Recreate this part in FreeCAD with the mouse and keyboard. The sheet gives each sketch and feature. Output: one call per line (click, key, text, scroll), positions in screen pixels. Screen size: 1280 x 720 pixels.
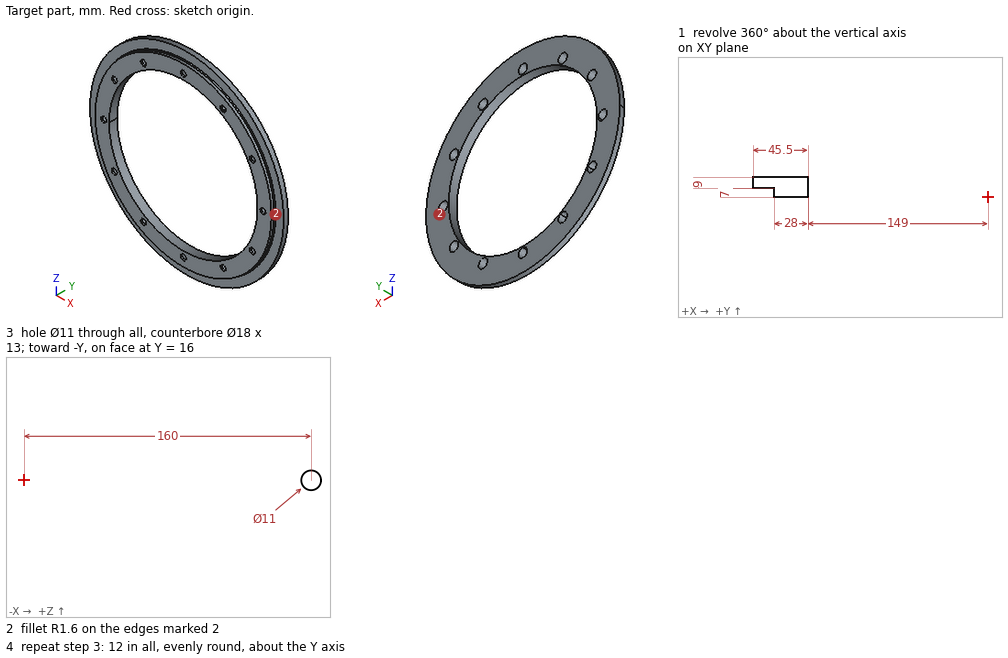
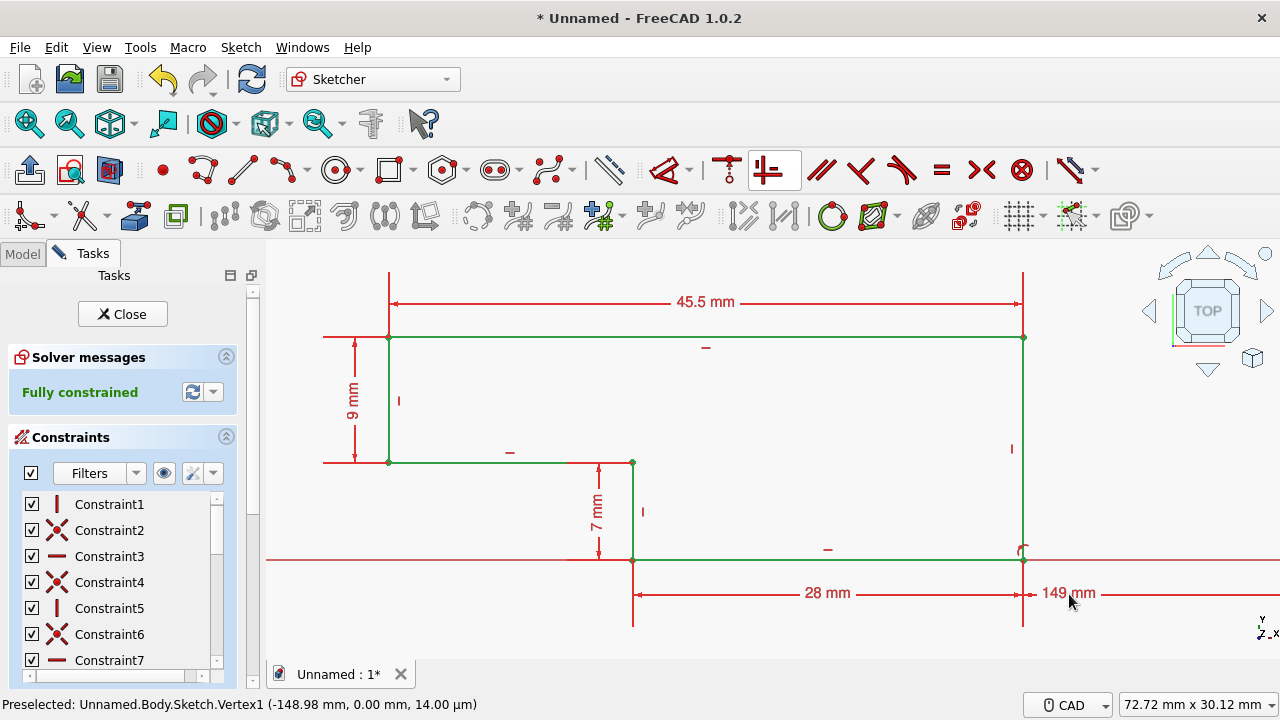
click(123, 314)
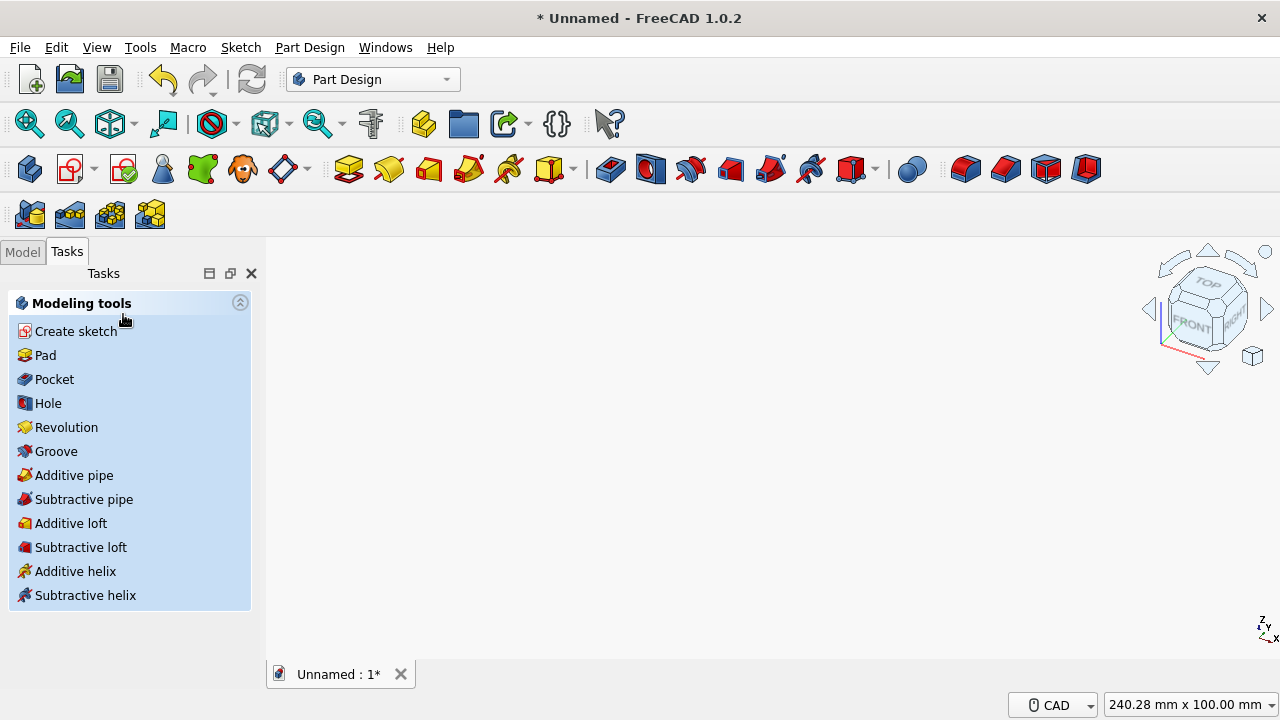
click(390, 170)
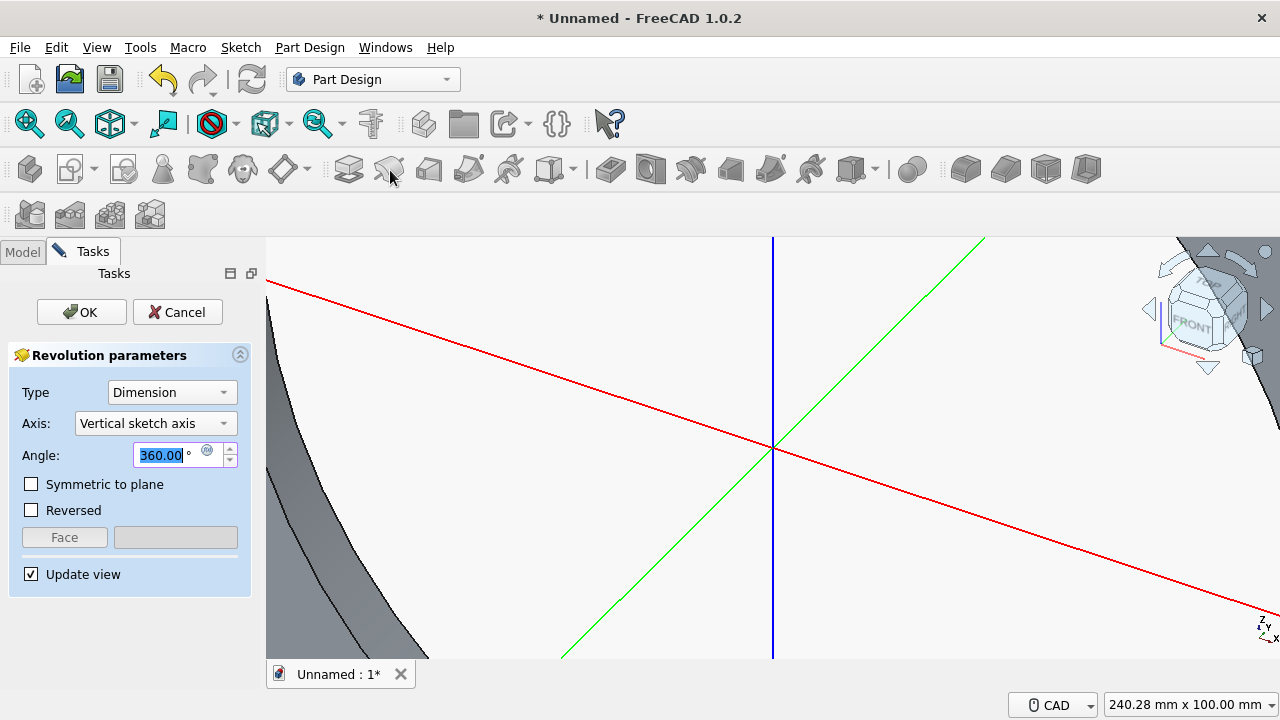
click(82, 312)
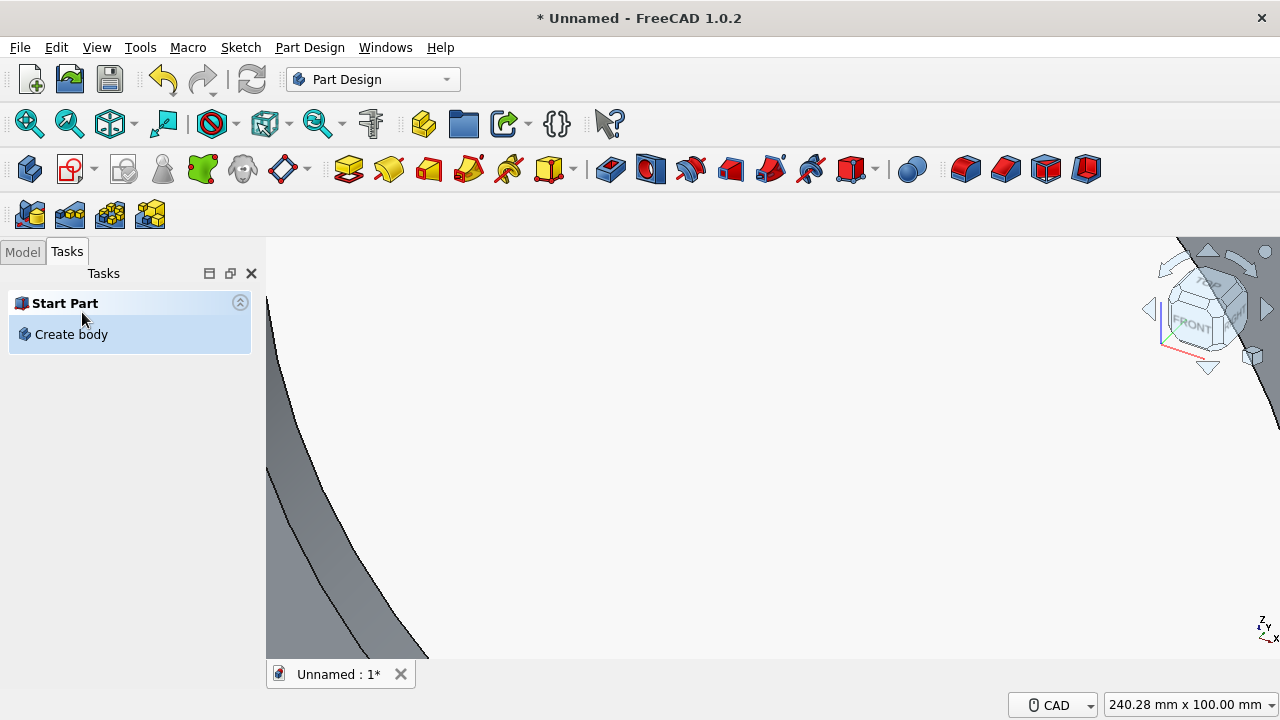
click(30, 124)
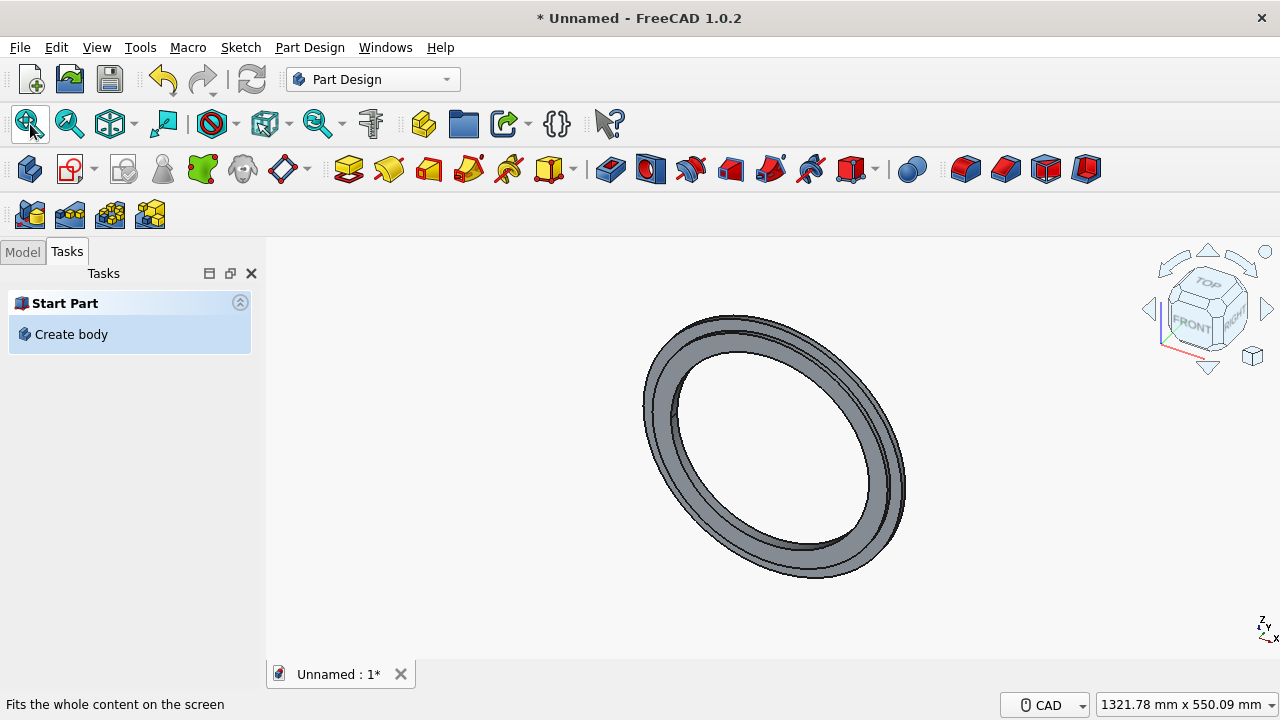
key(0)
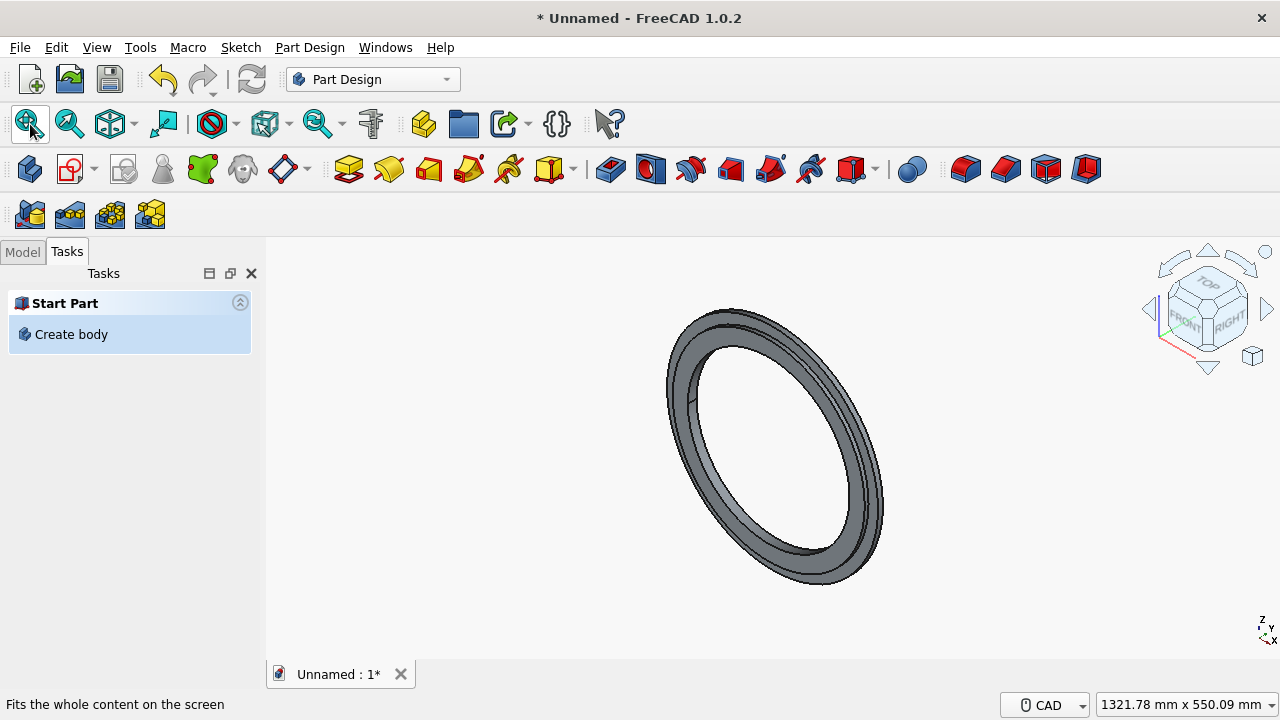
key(2)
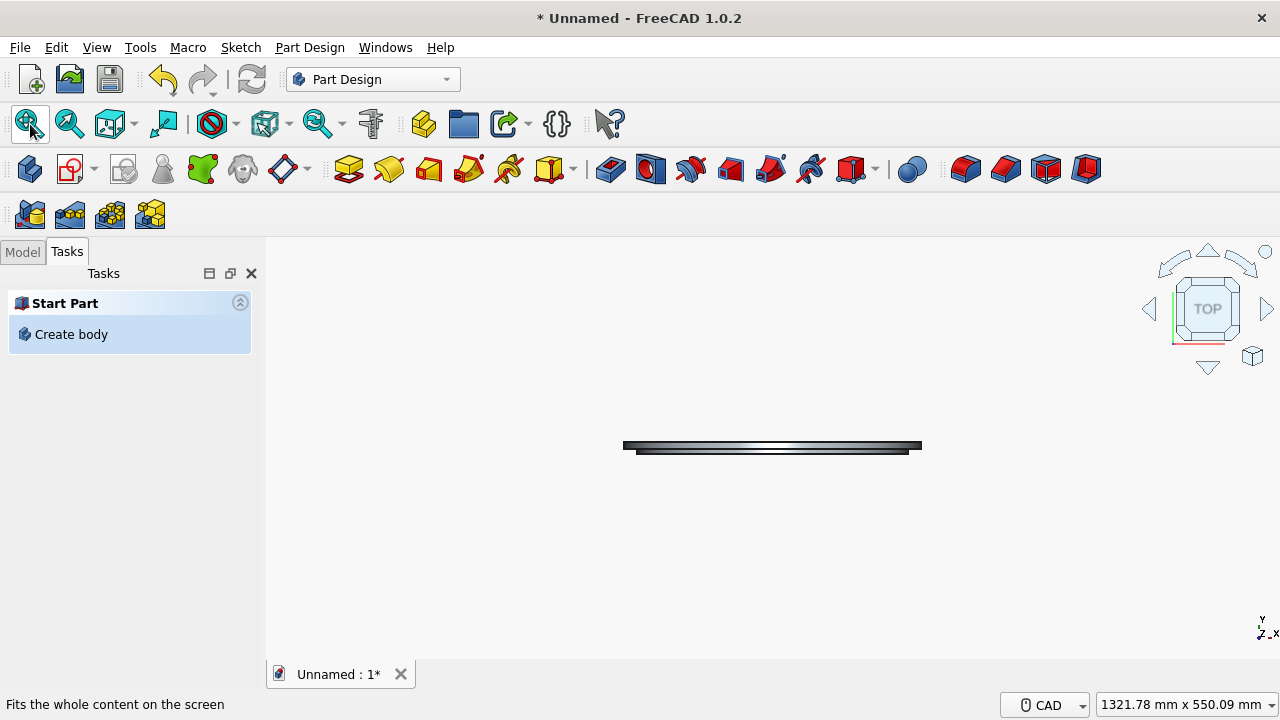
click(30, 124)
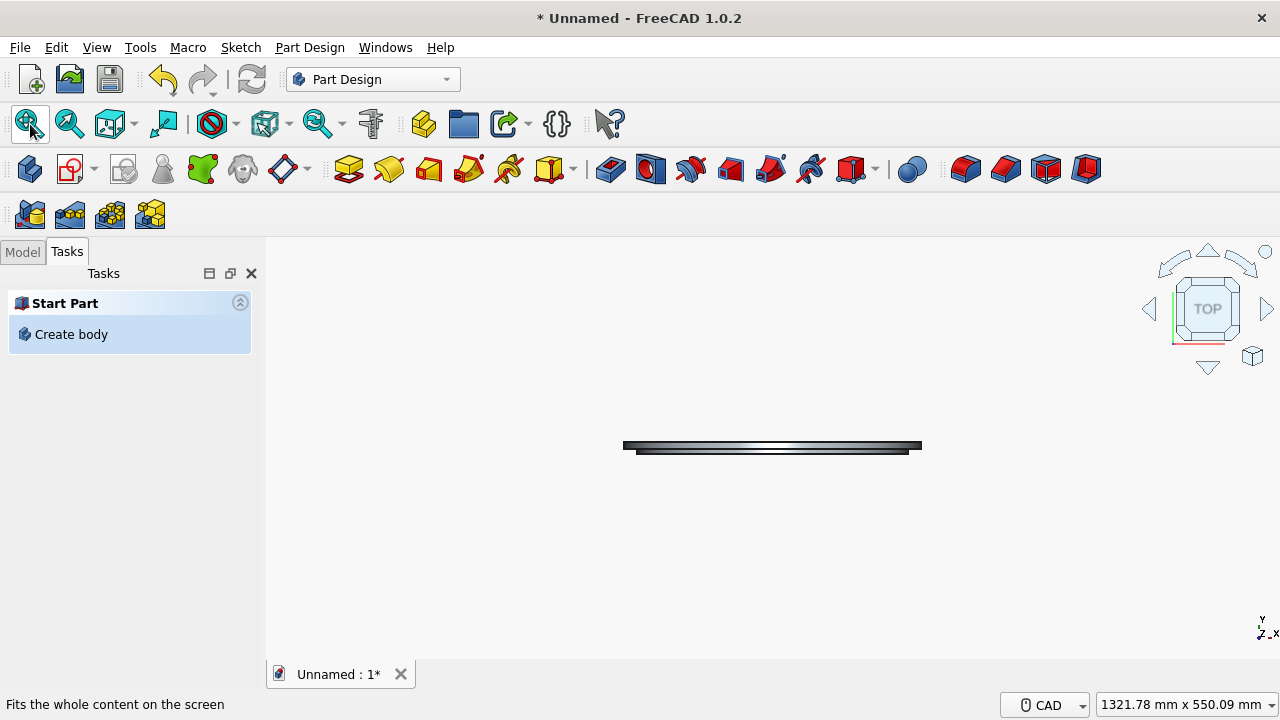
key(1)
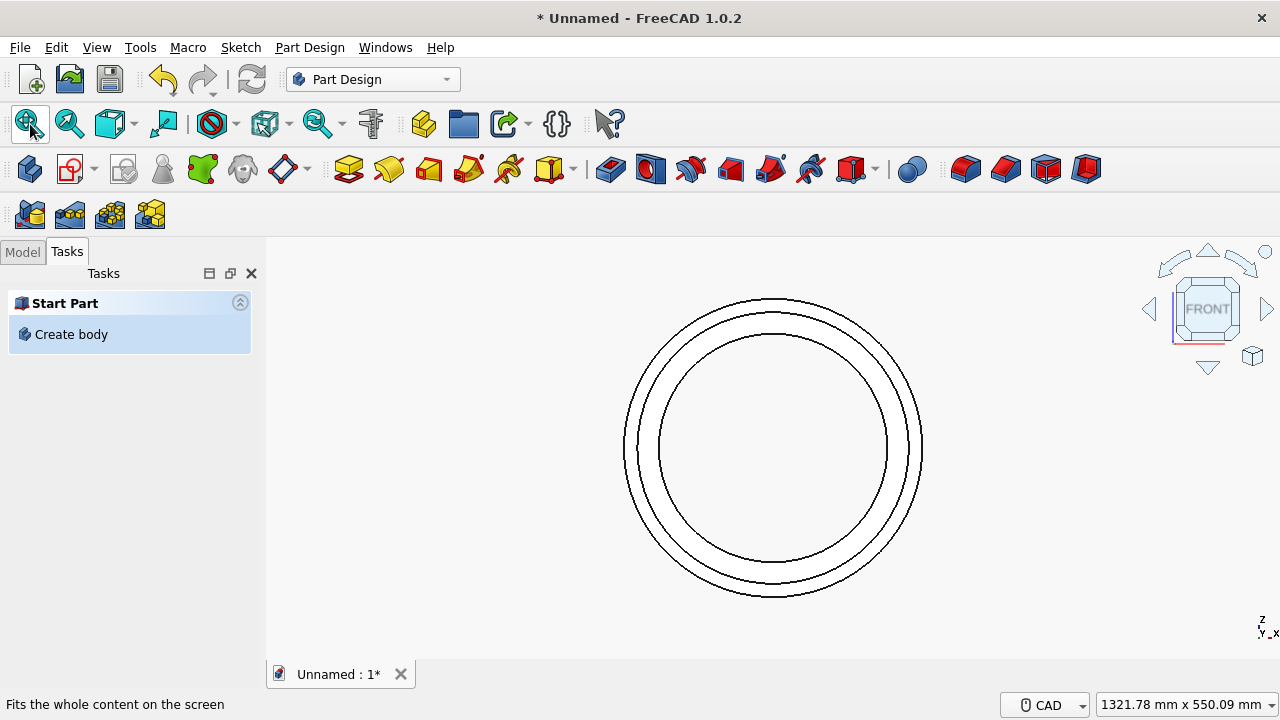
key(3)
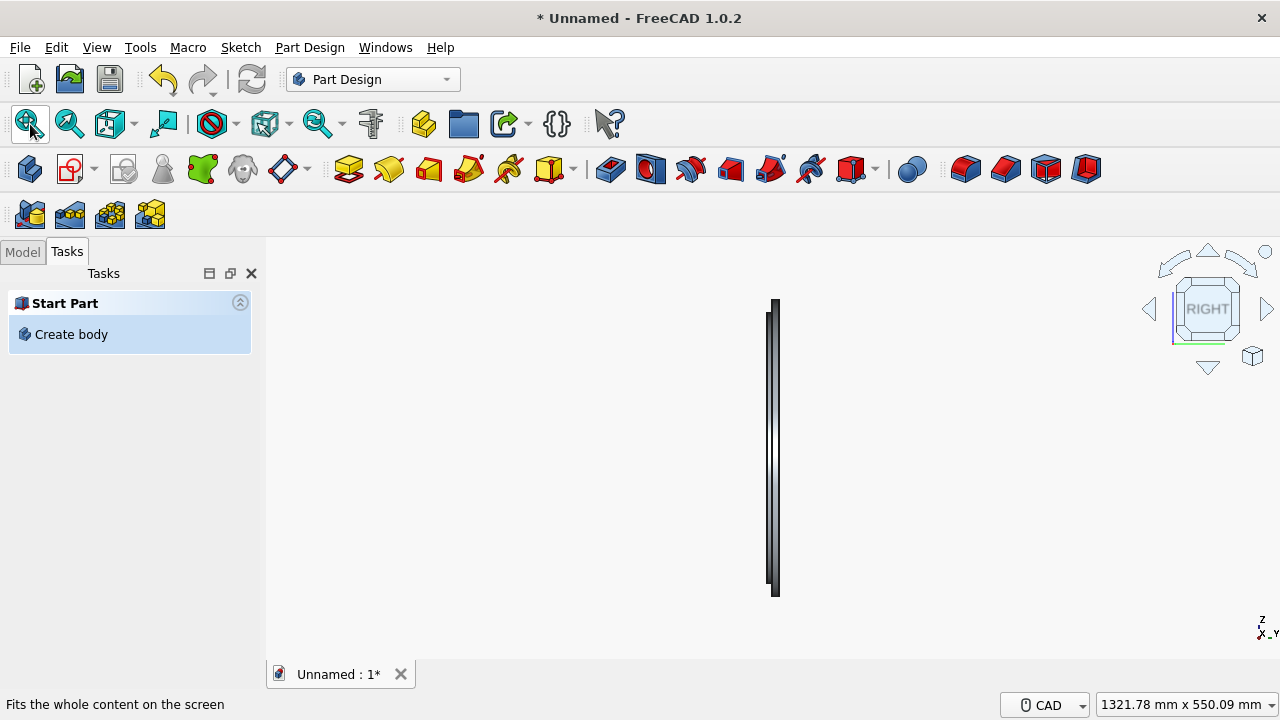
key(5)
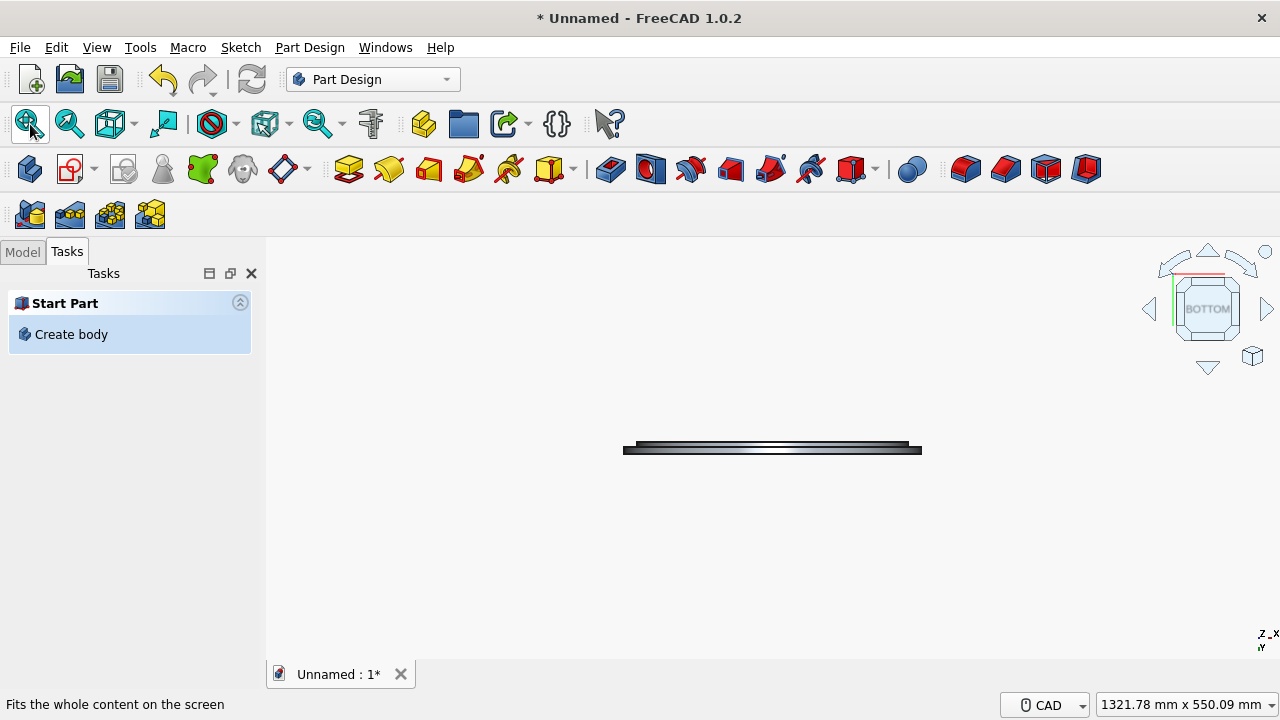
click(30, 124)